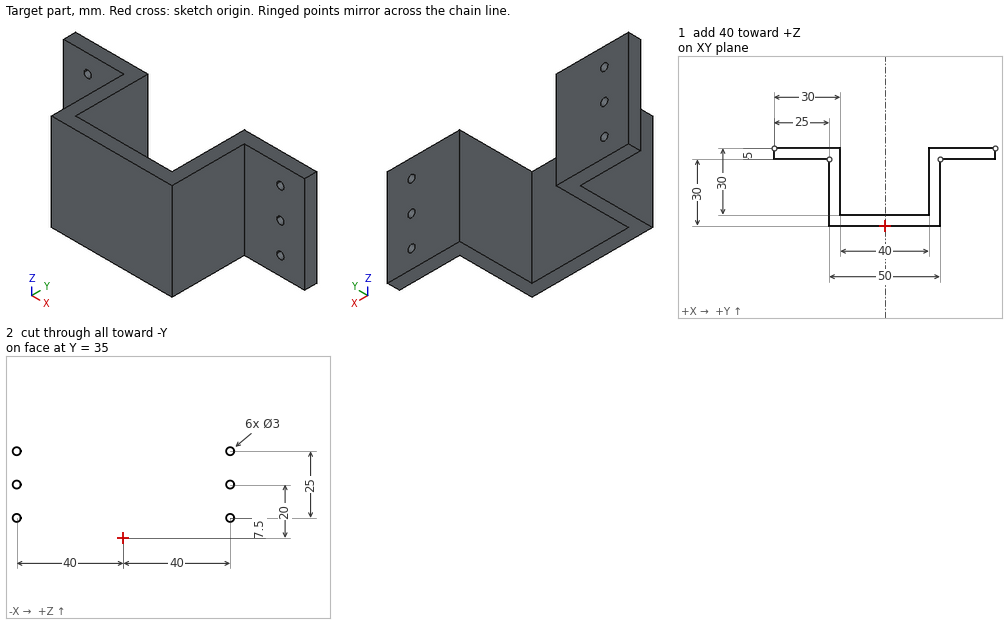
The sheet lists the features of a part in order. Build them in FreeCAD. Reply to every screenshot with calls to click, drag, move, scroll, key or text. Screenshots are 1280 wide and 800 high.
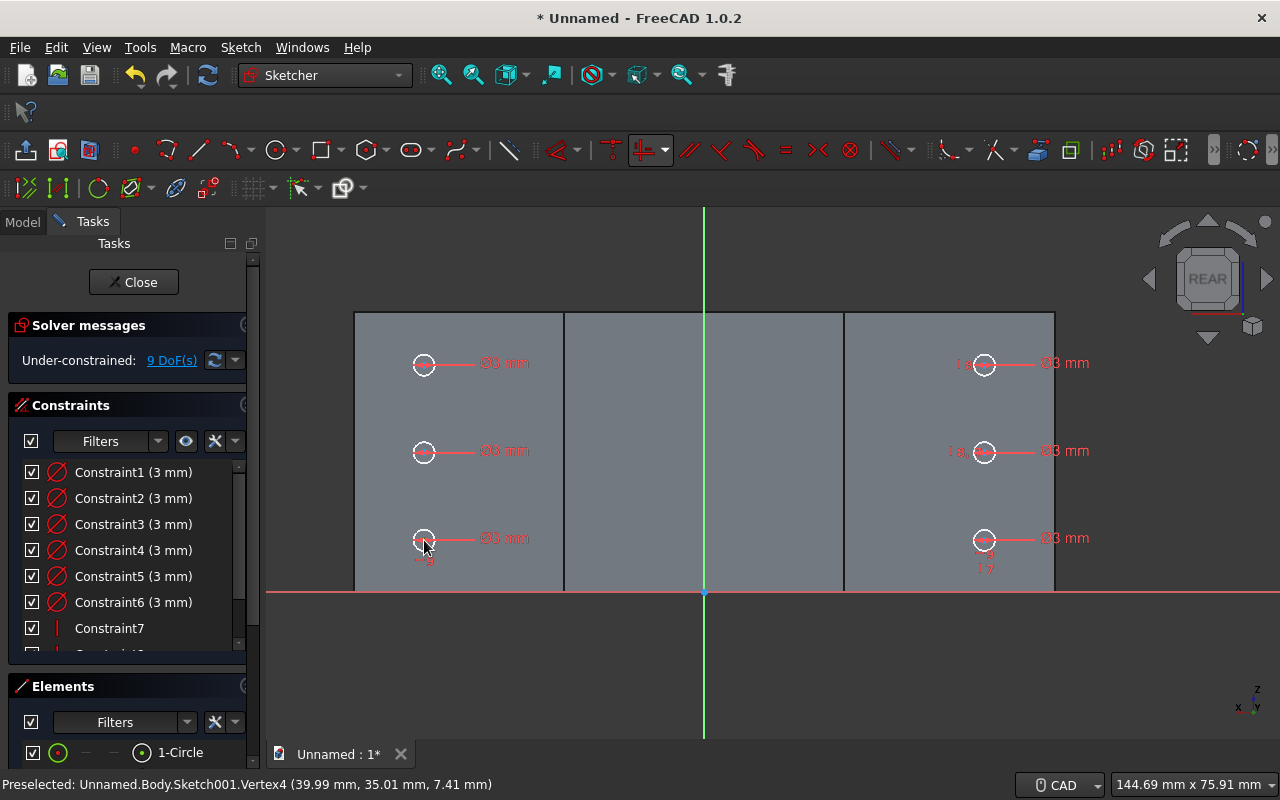
click(424, 453)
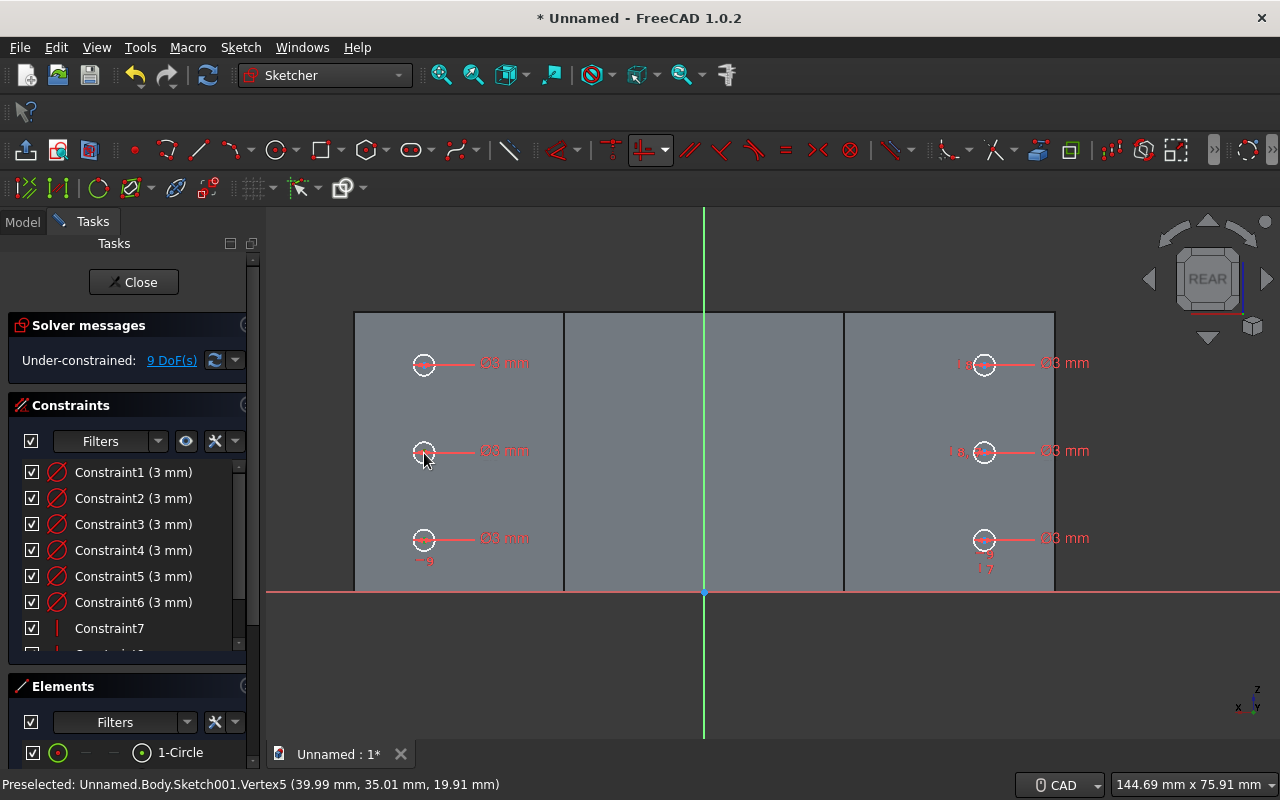
key(v)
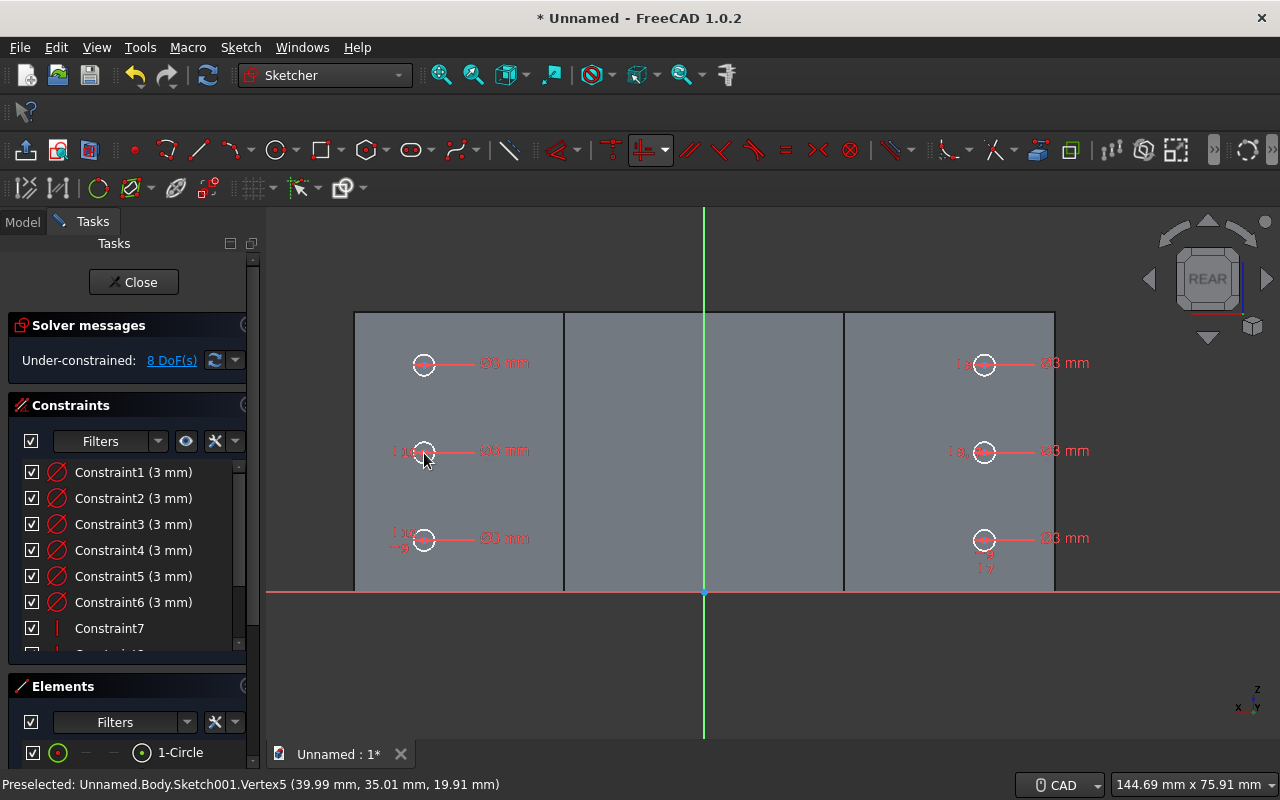
click(984, 453)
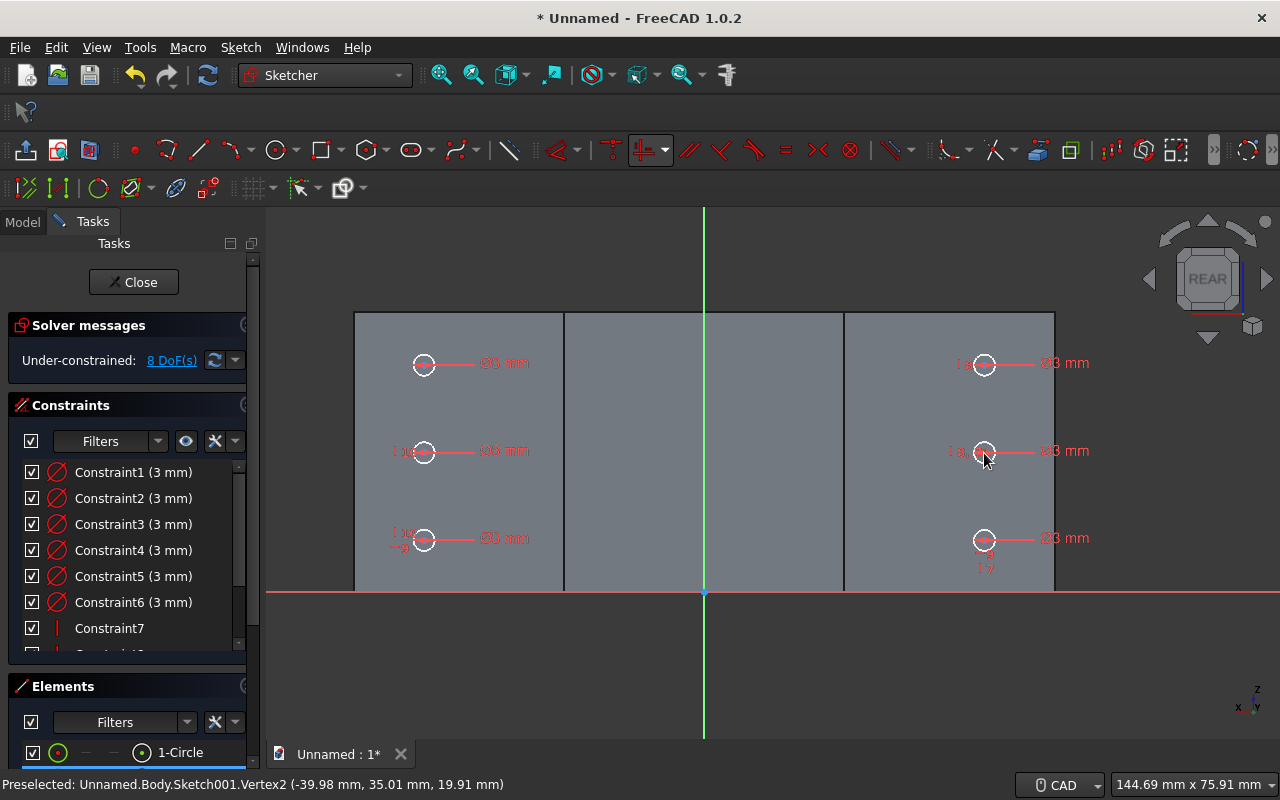
click(424, 453)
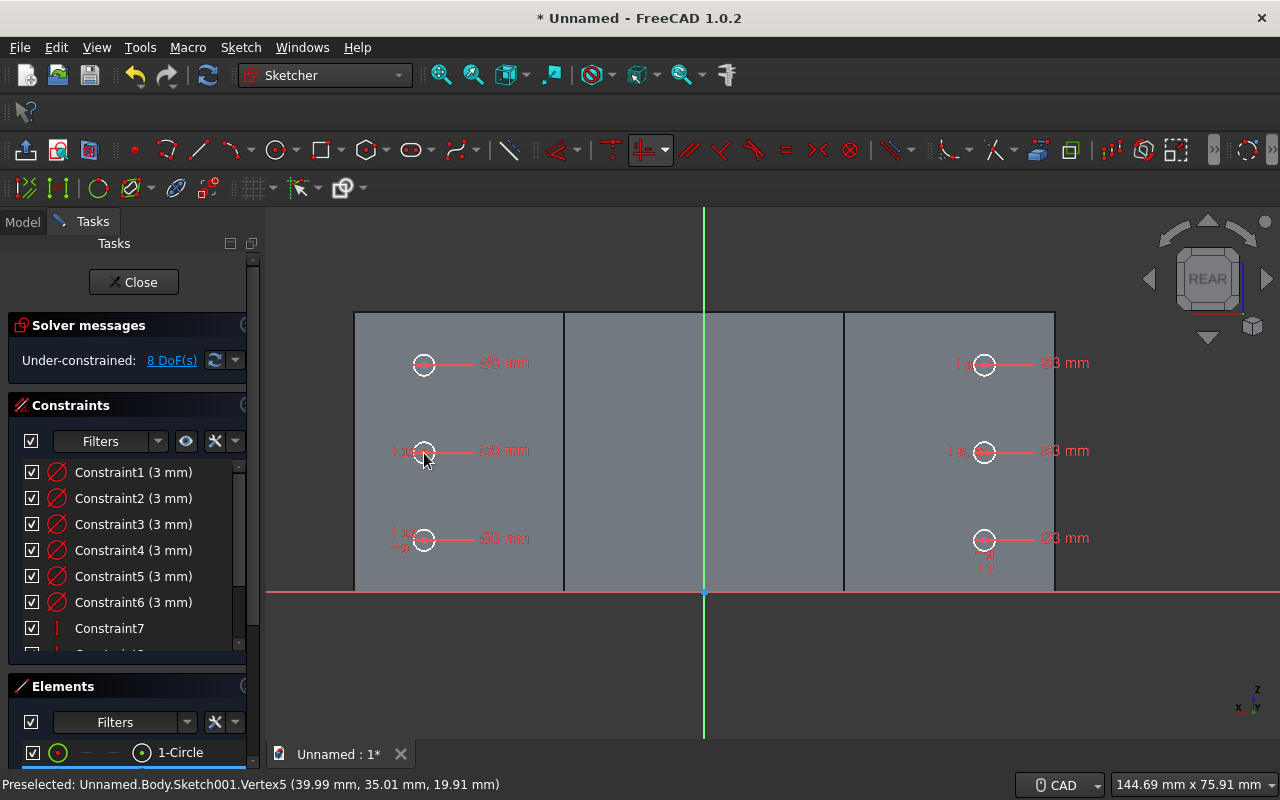
key(h)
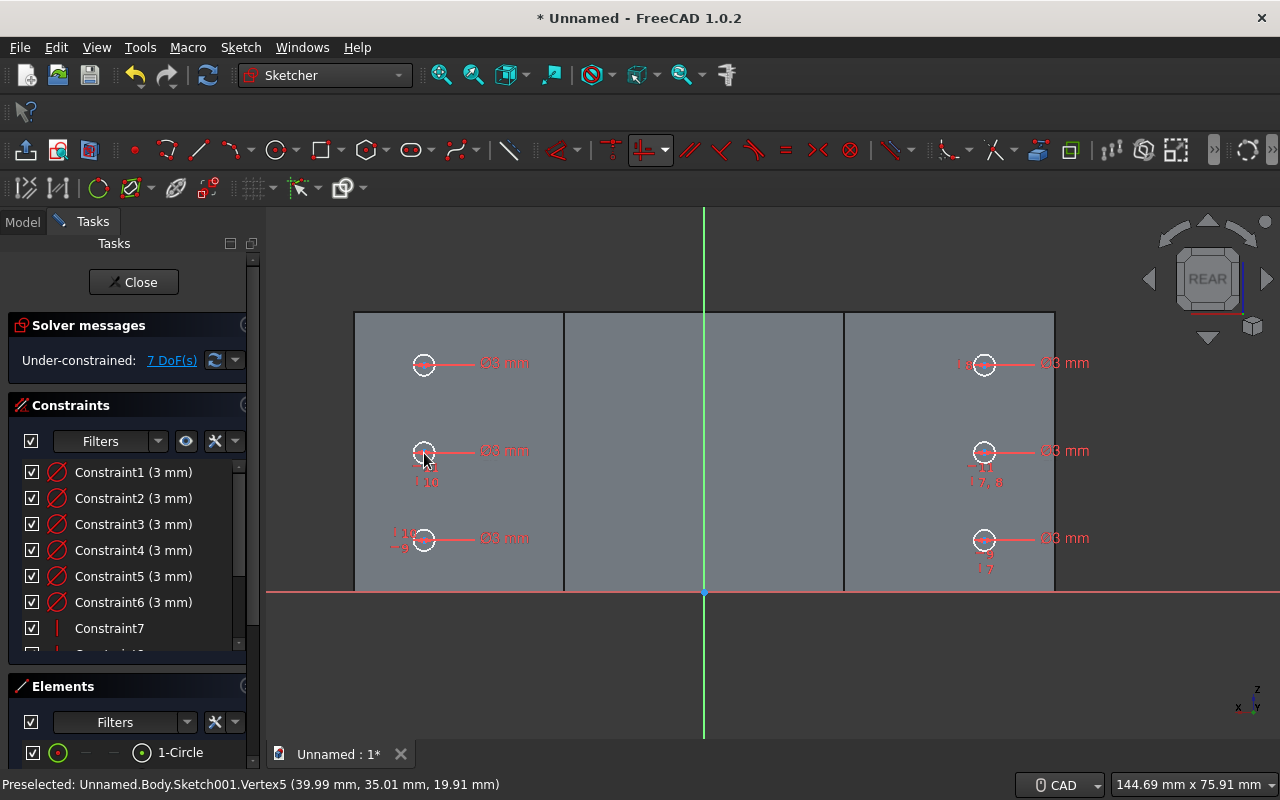
click(424, 453)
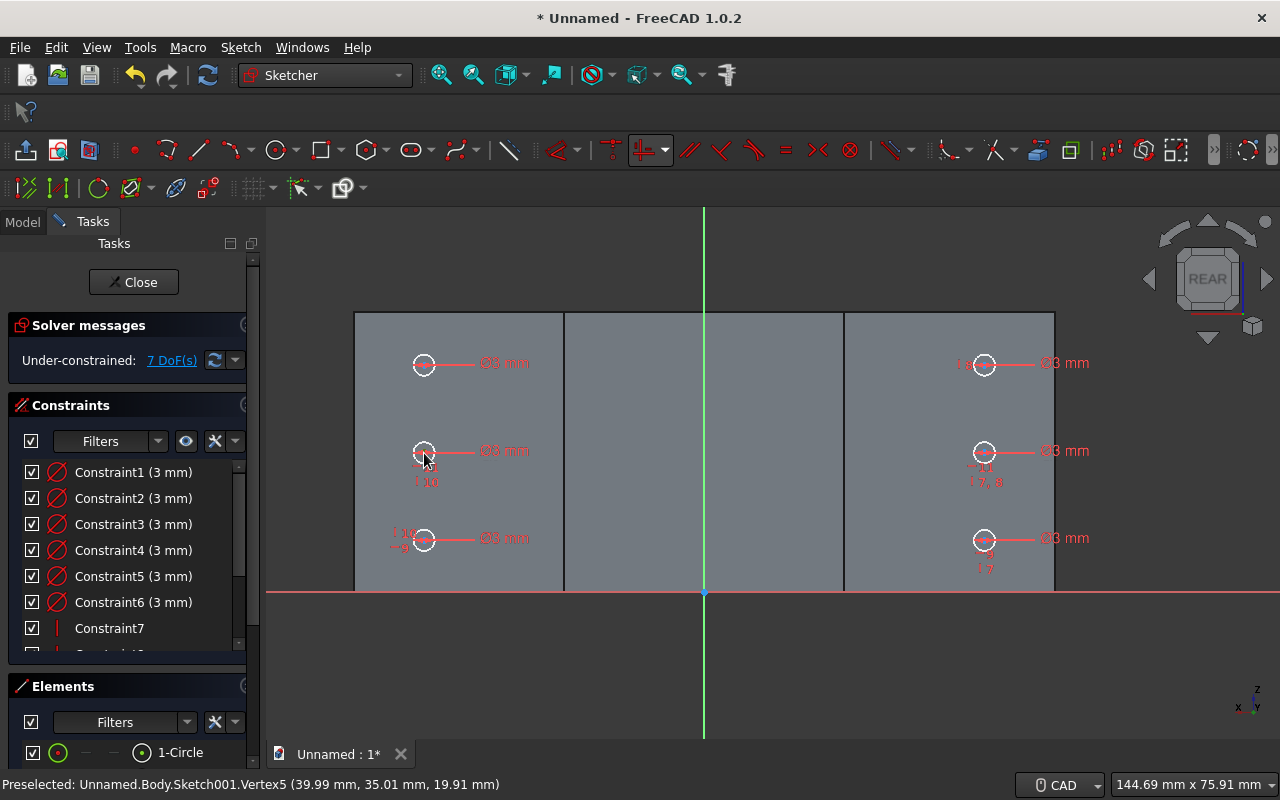
click(424, 365)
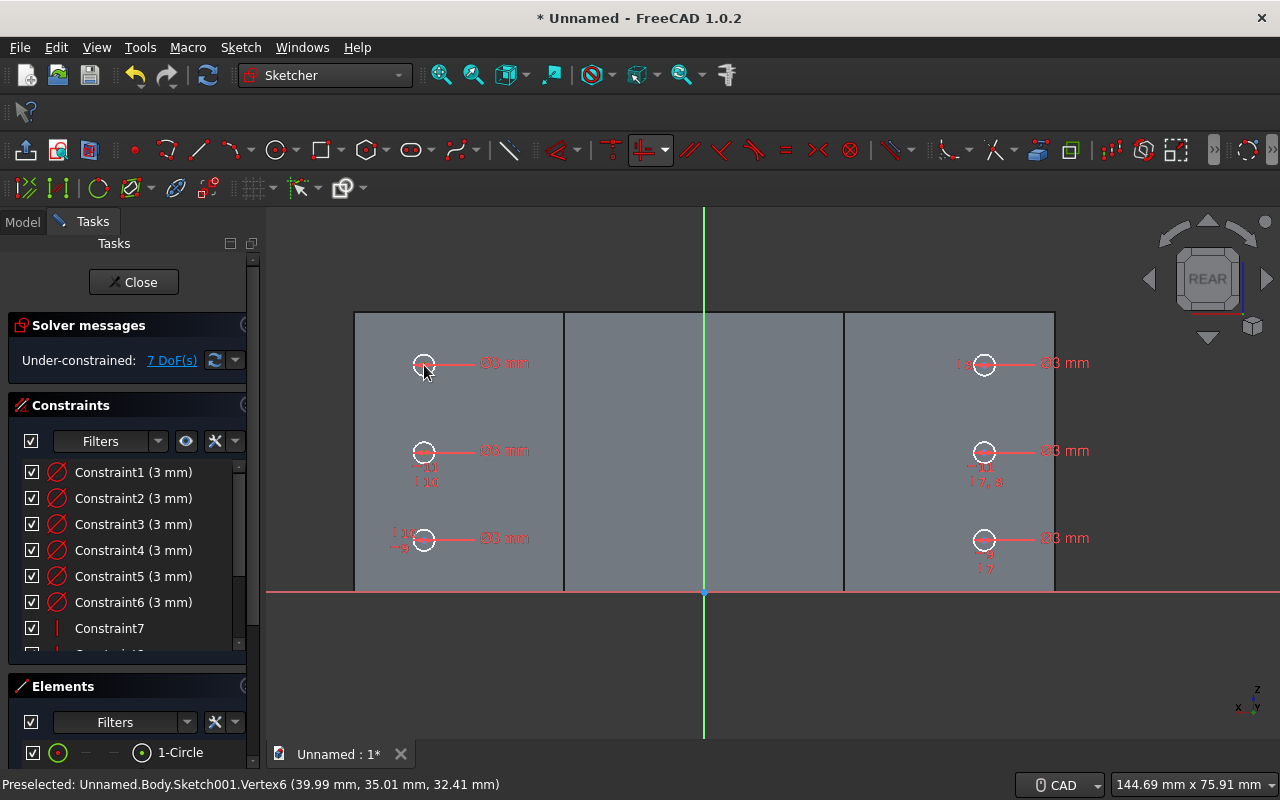
key(v)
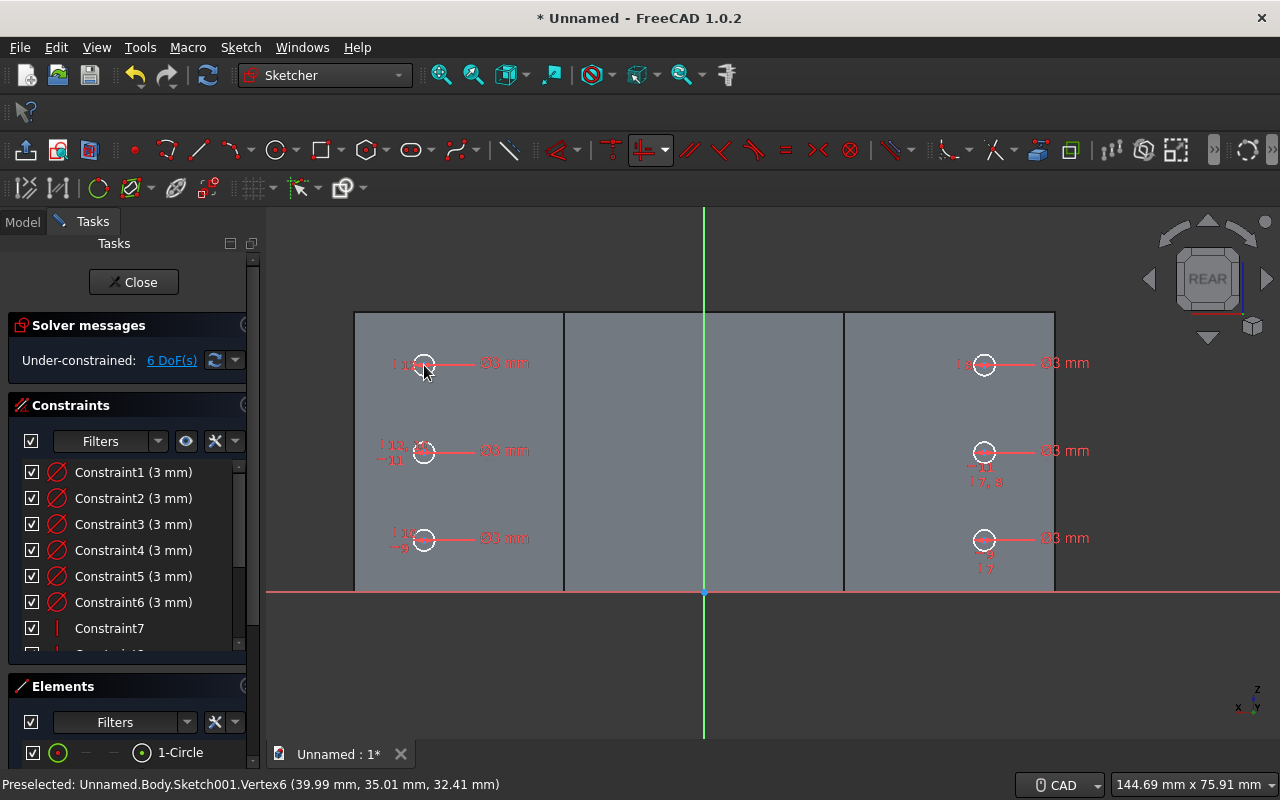
click(984, 365)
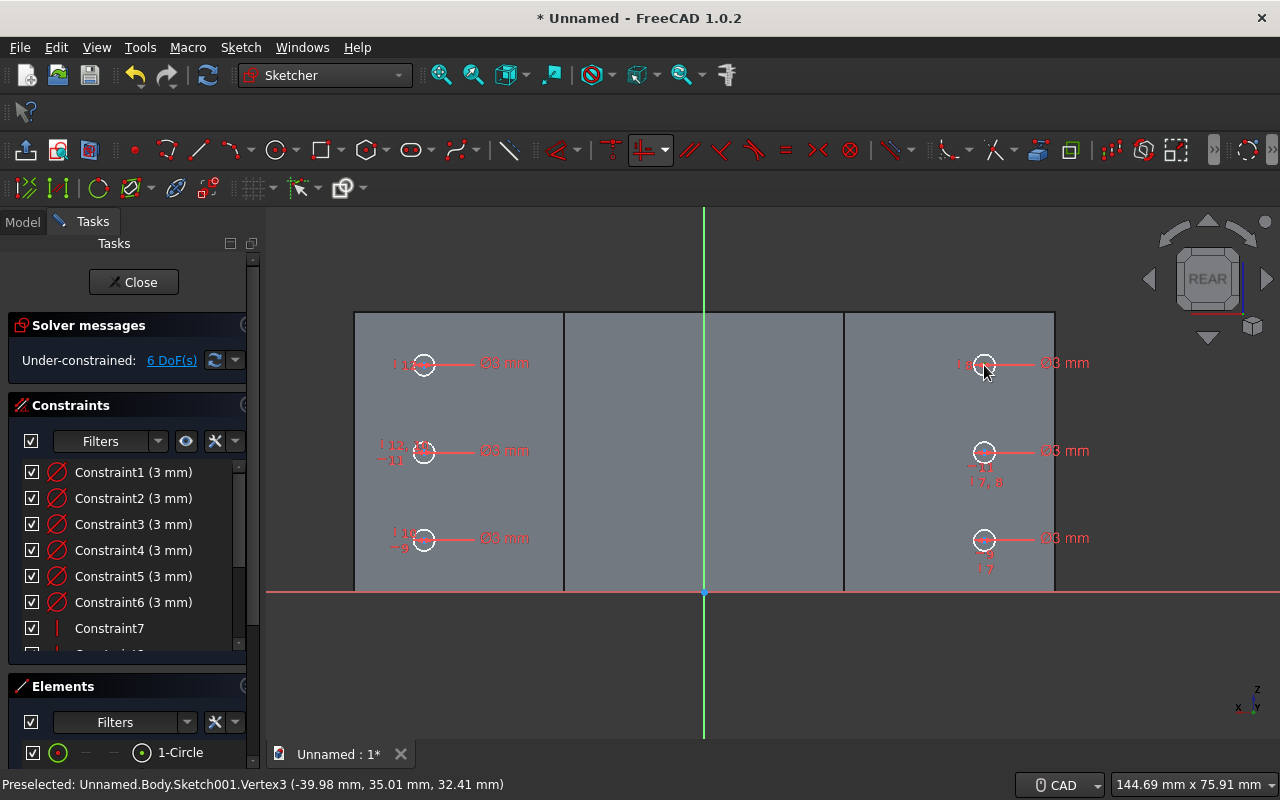
click(424, 365)